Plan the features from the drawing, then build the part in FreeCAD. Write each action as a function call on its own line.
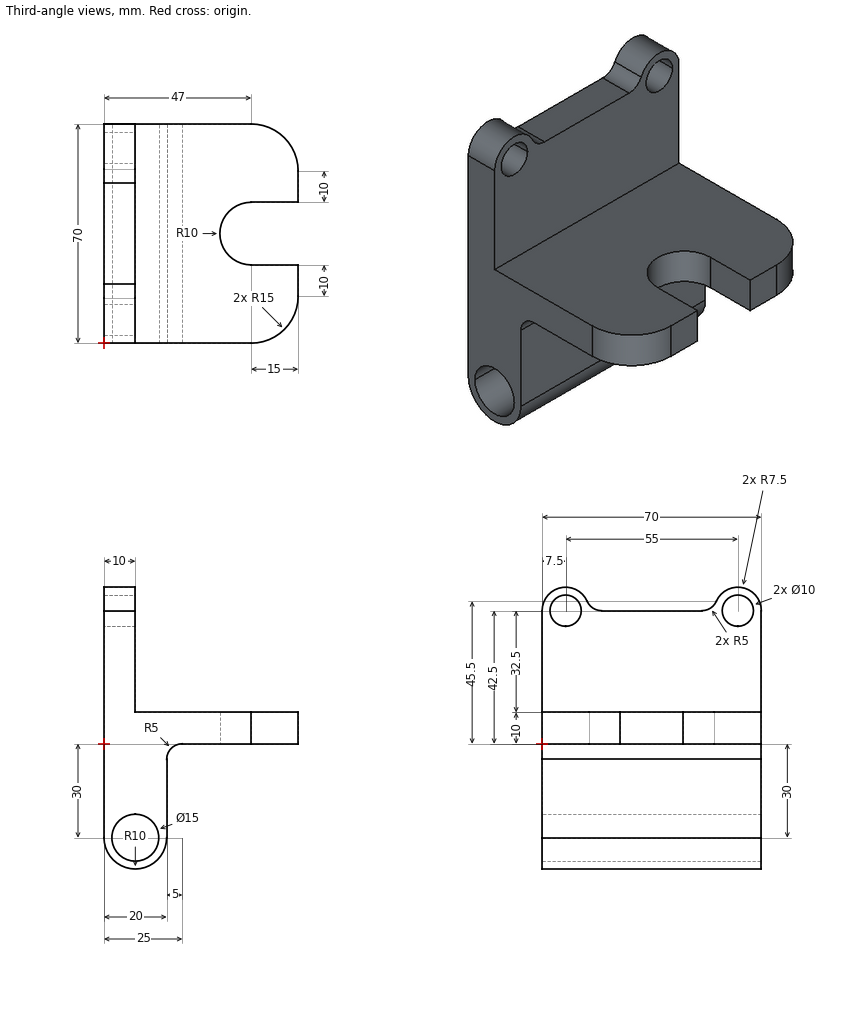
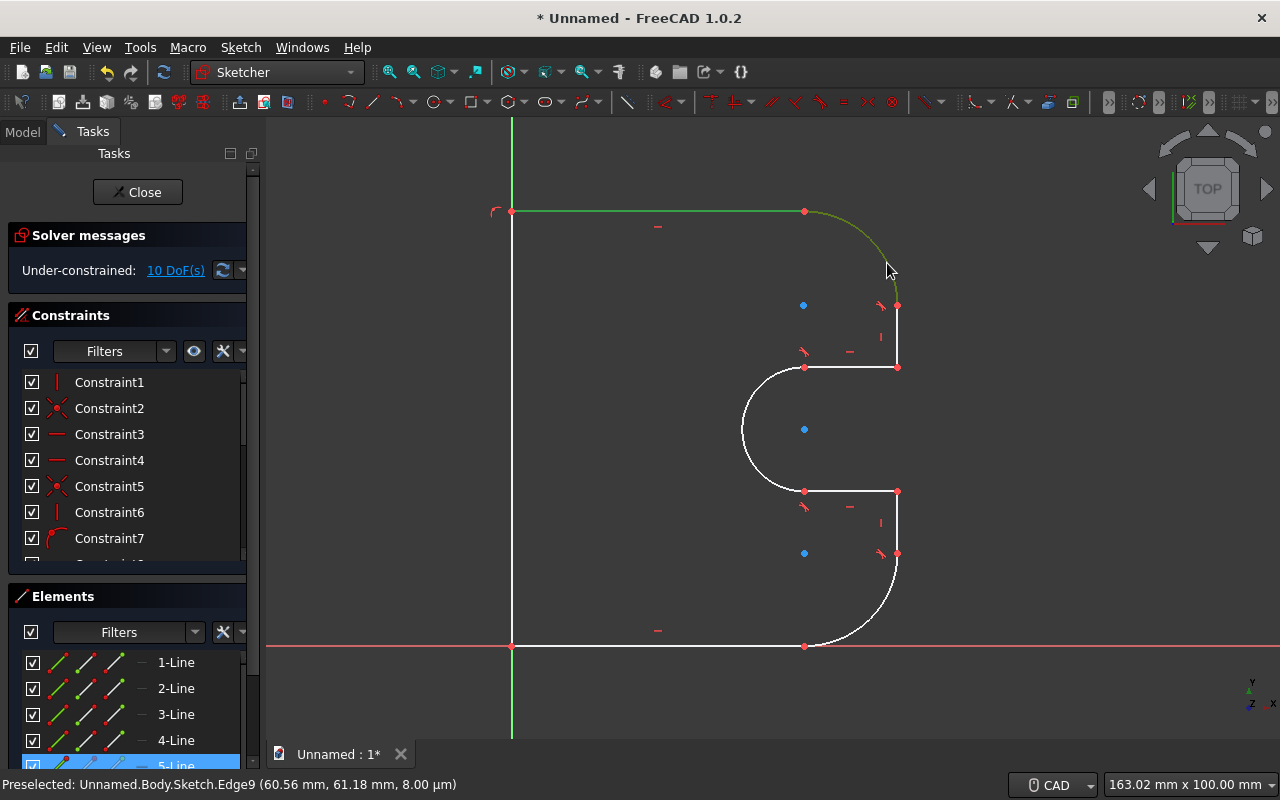
click(820, 102)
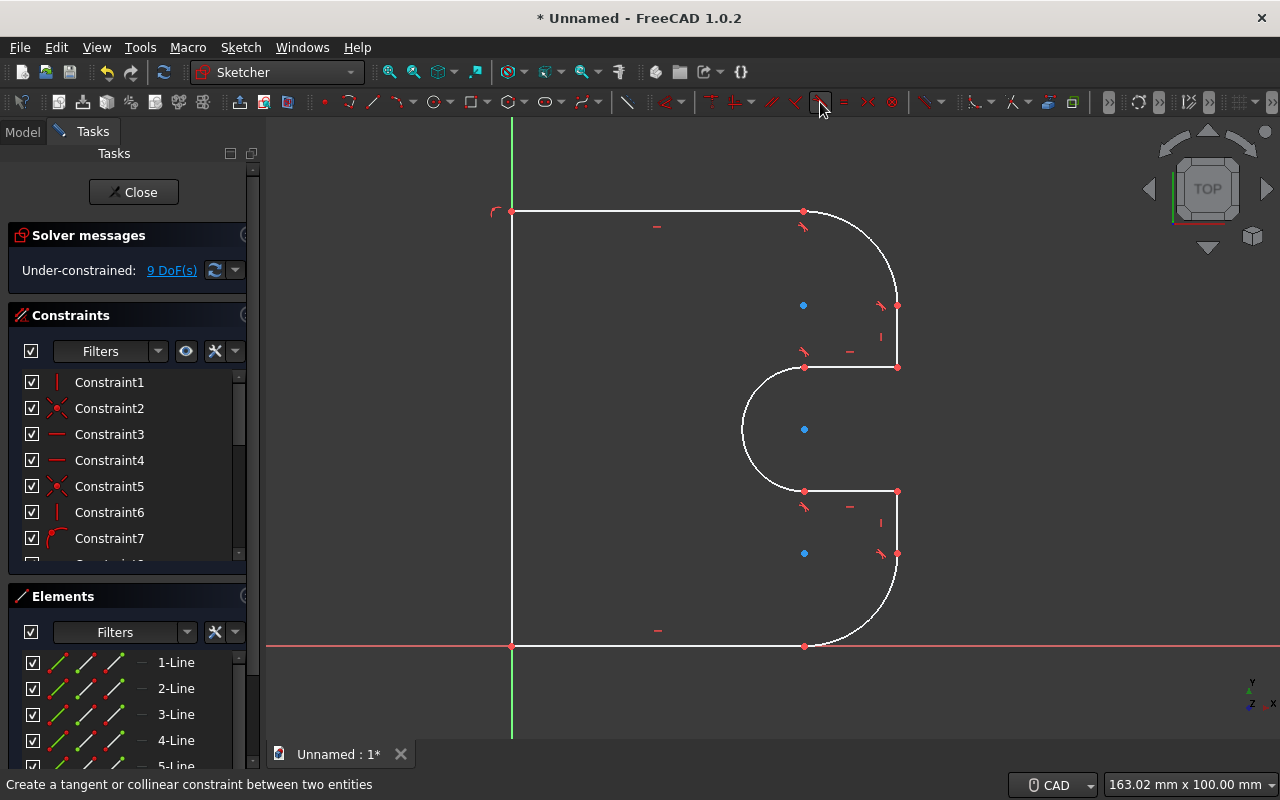
click(600, 646)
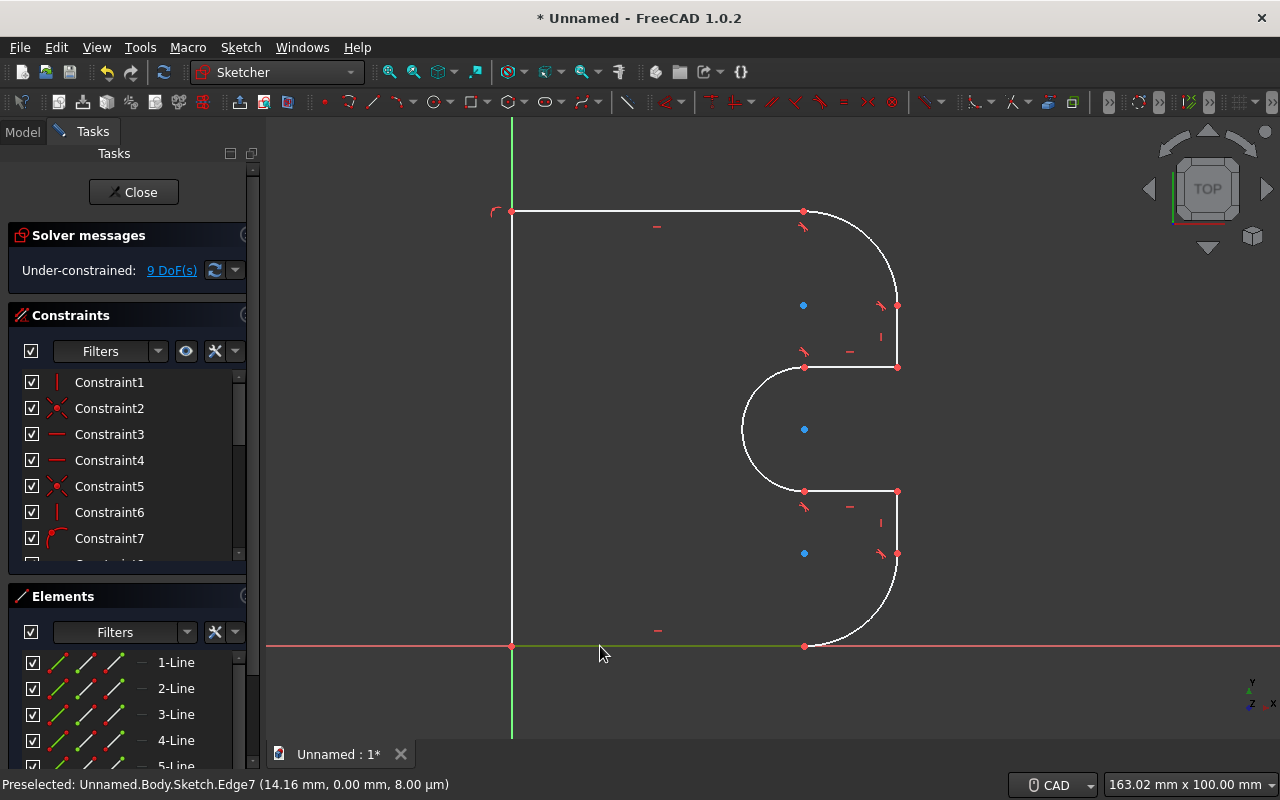
scroll(847, 636, up, 2)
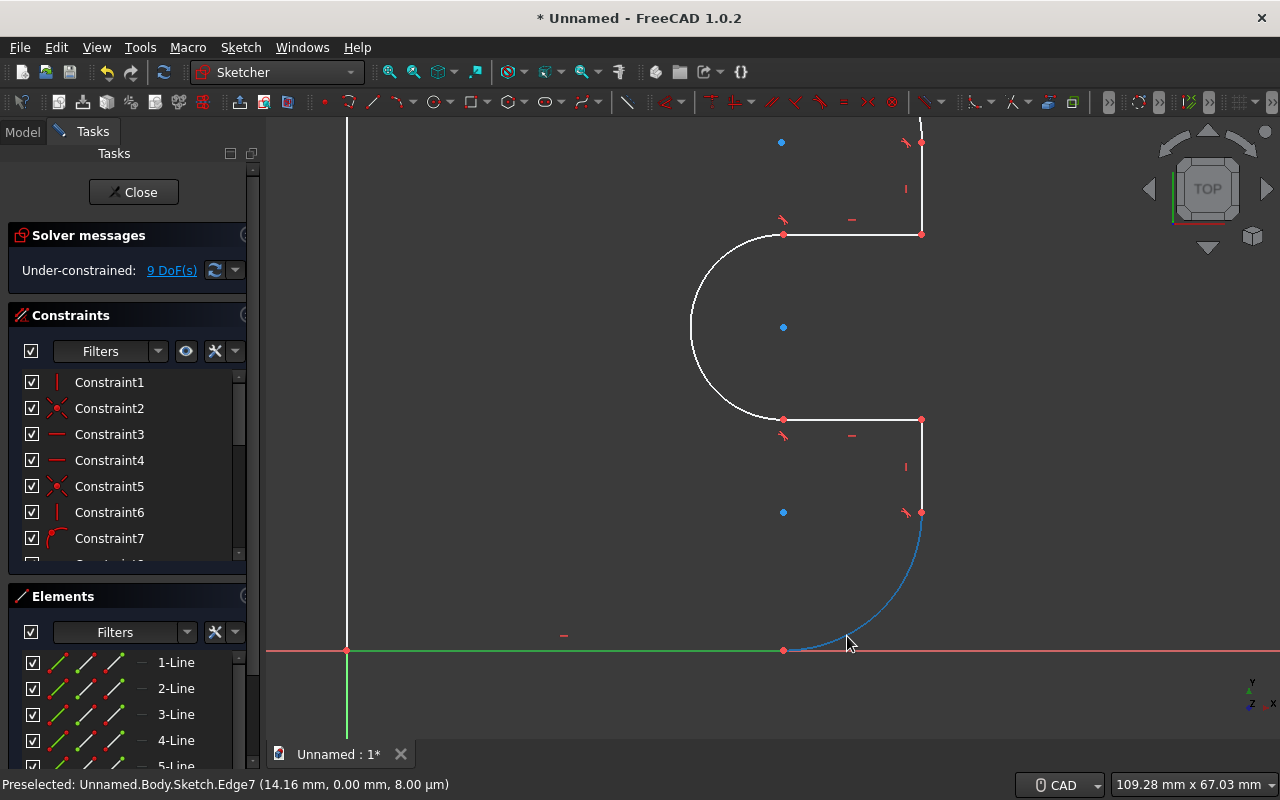
click(846, 636)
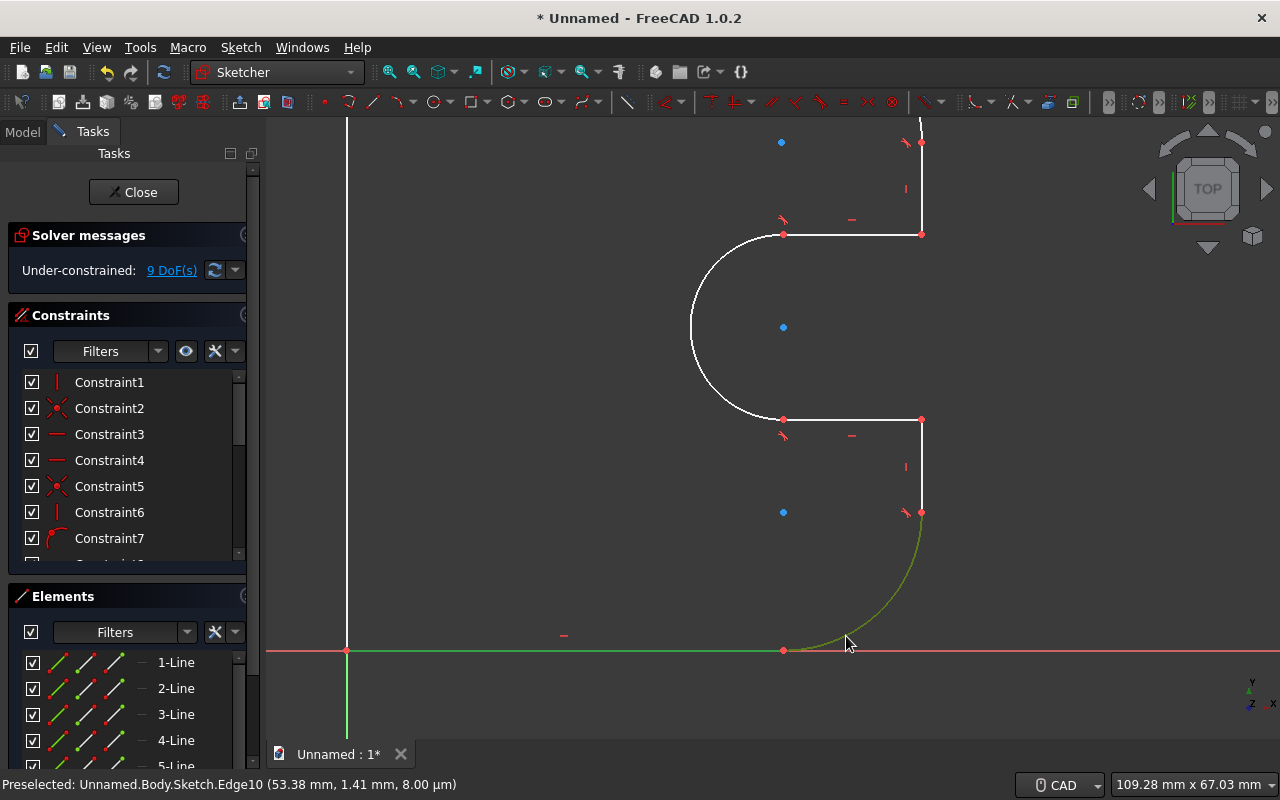
click(820, 102)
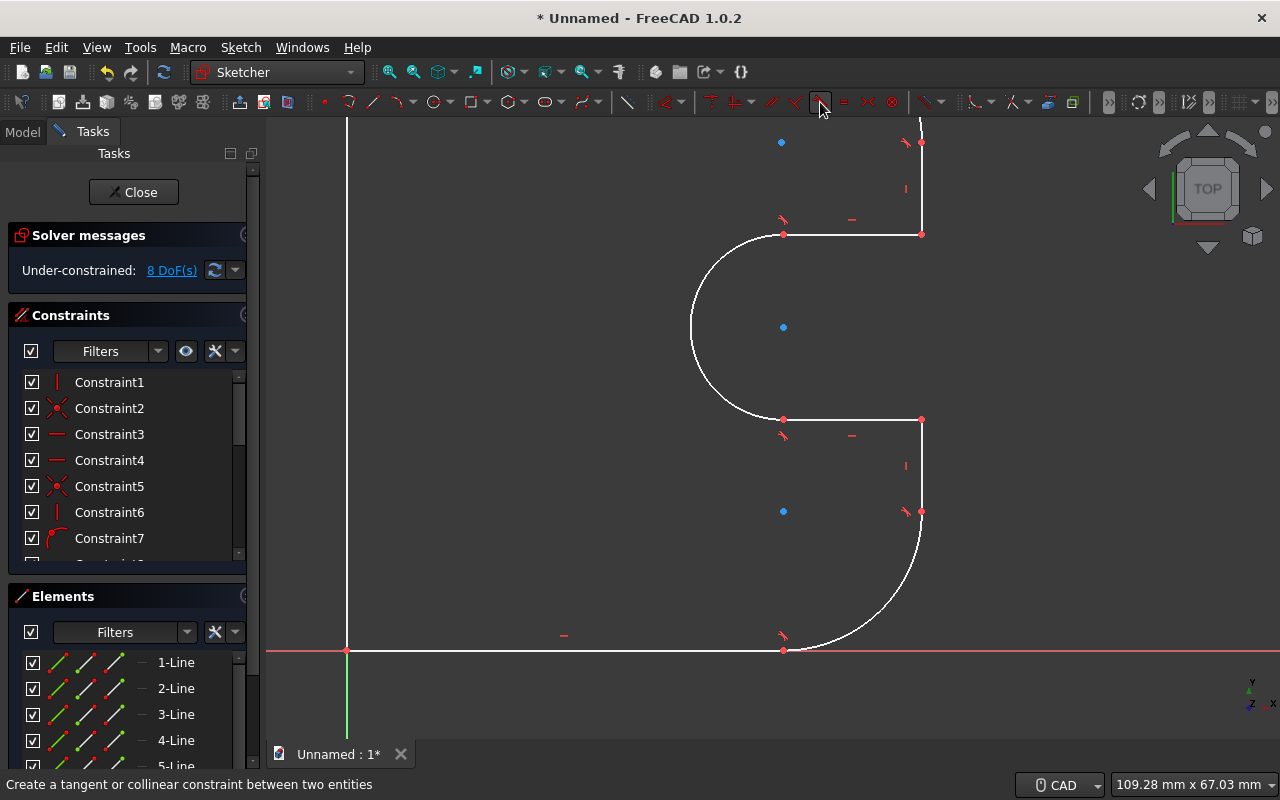
scroll(847, 636, down, 2)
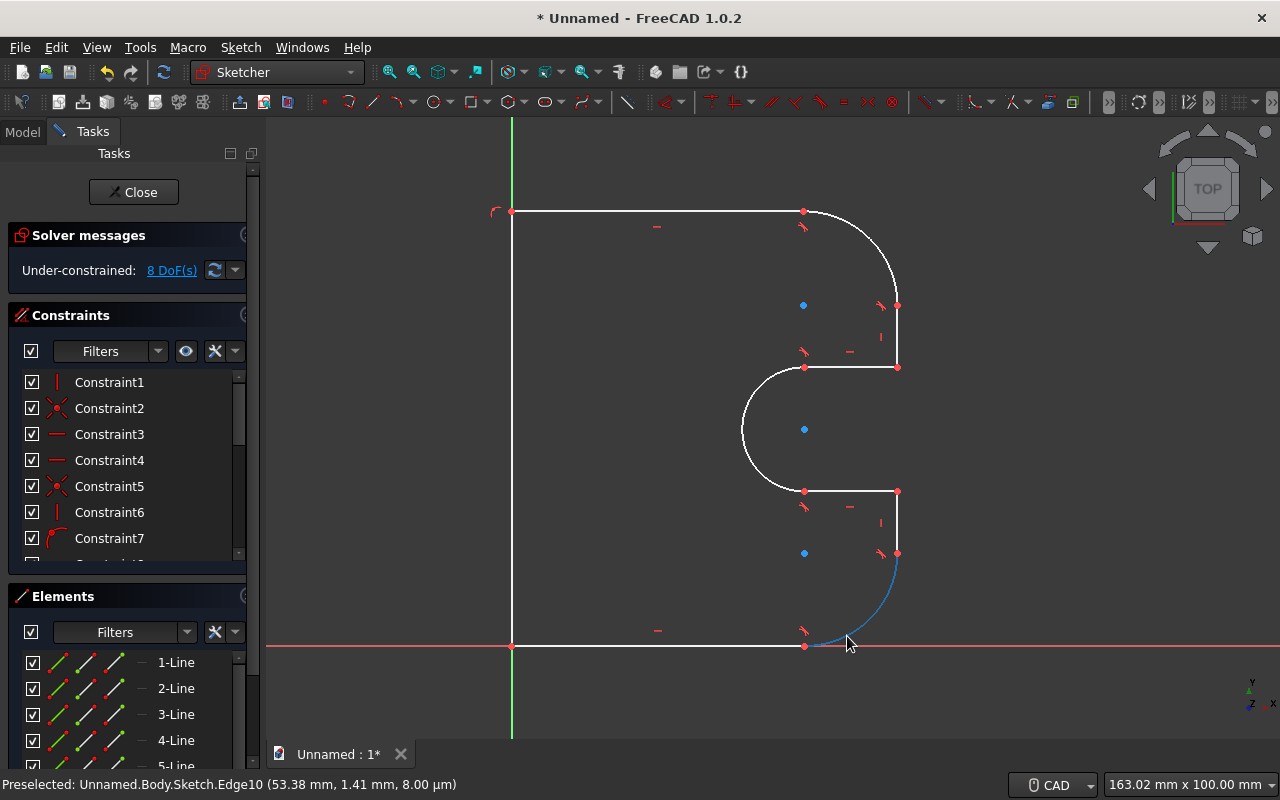
click(887, 263)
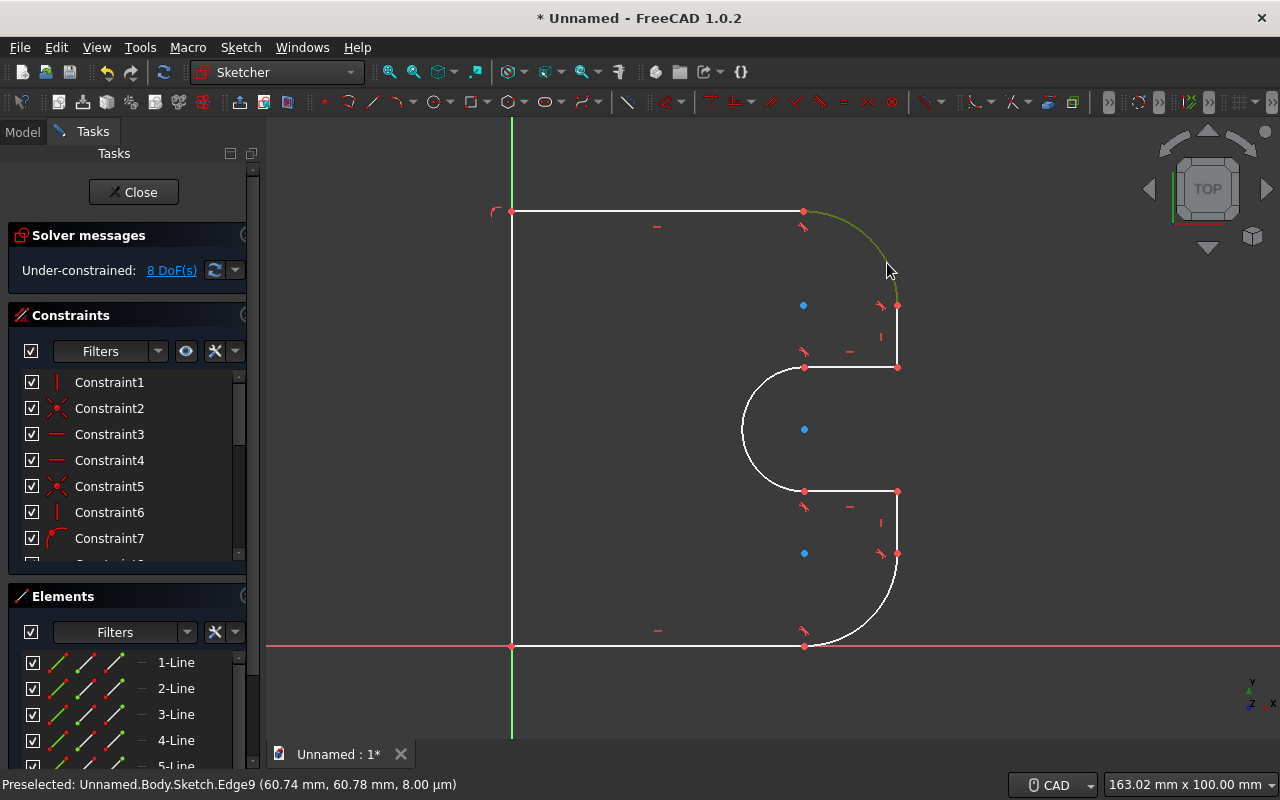
scroll(847, 636, up, 2)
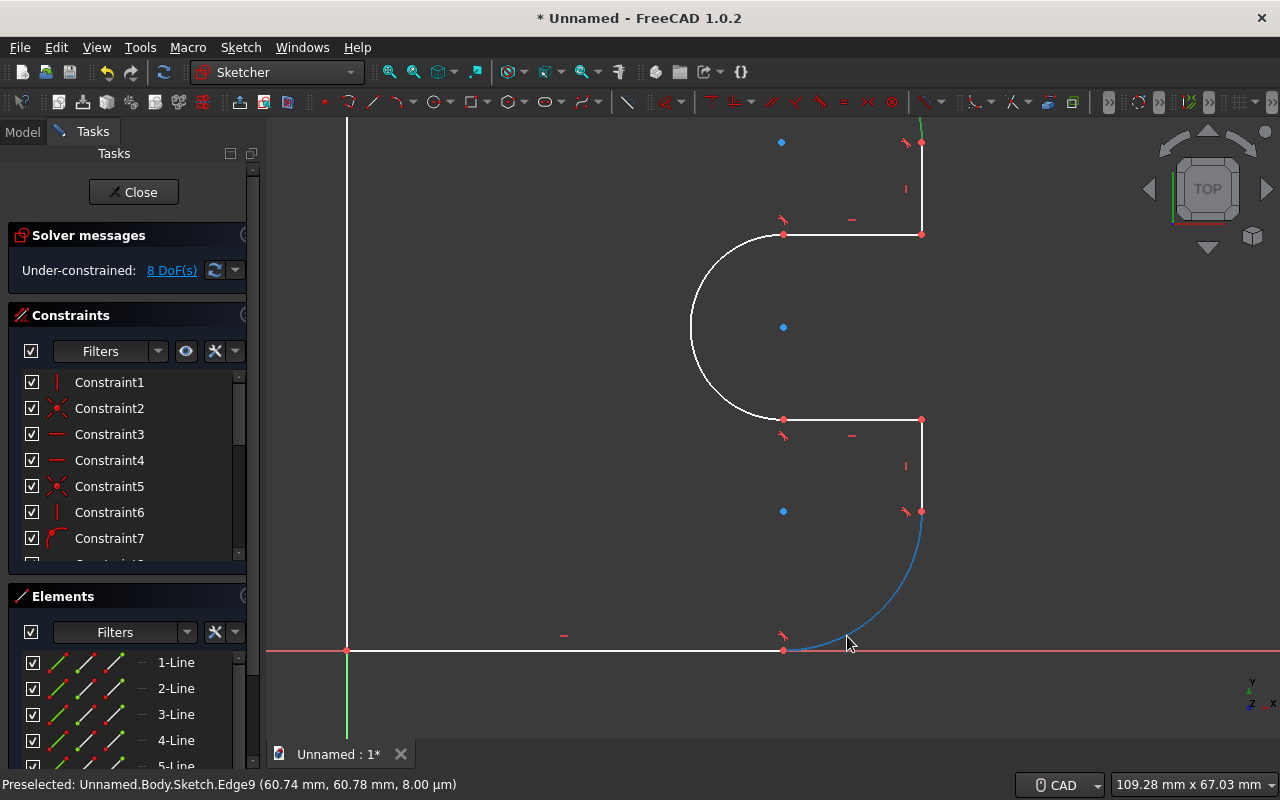
click(846, 635)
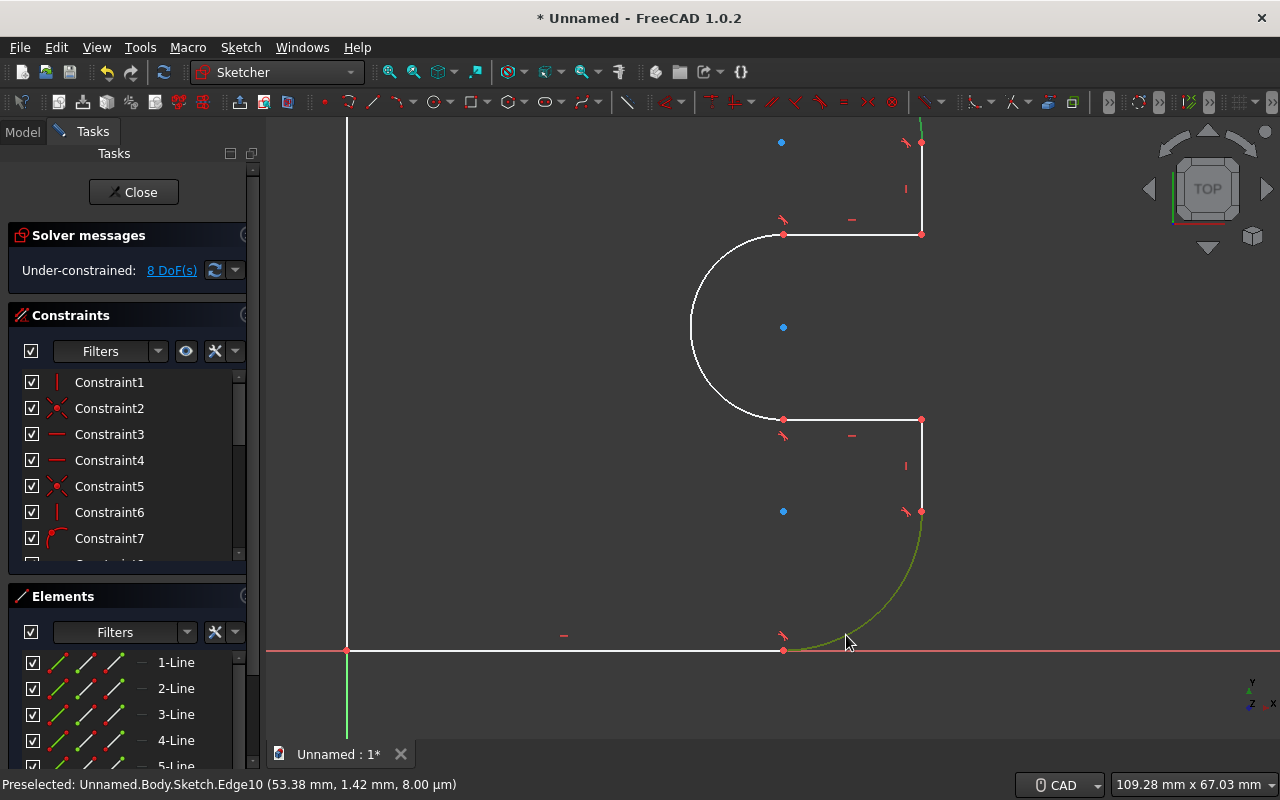
click(844, 102)